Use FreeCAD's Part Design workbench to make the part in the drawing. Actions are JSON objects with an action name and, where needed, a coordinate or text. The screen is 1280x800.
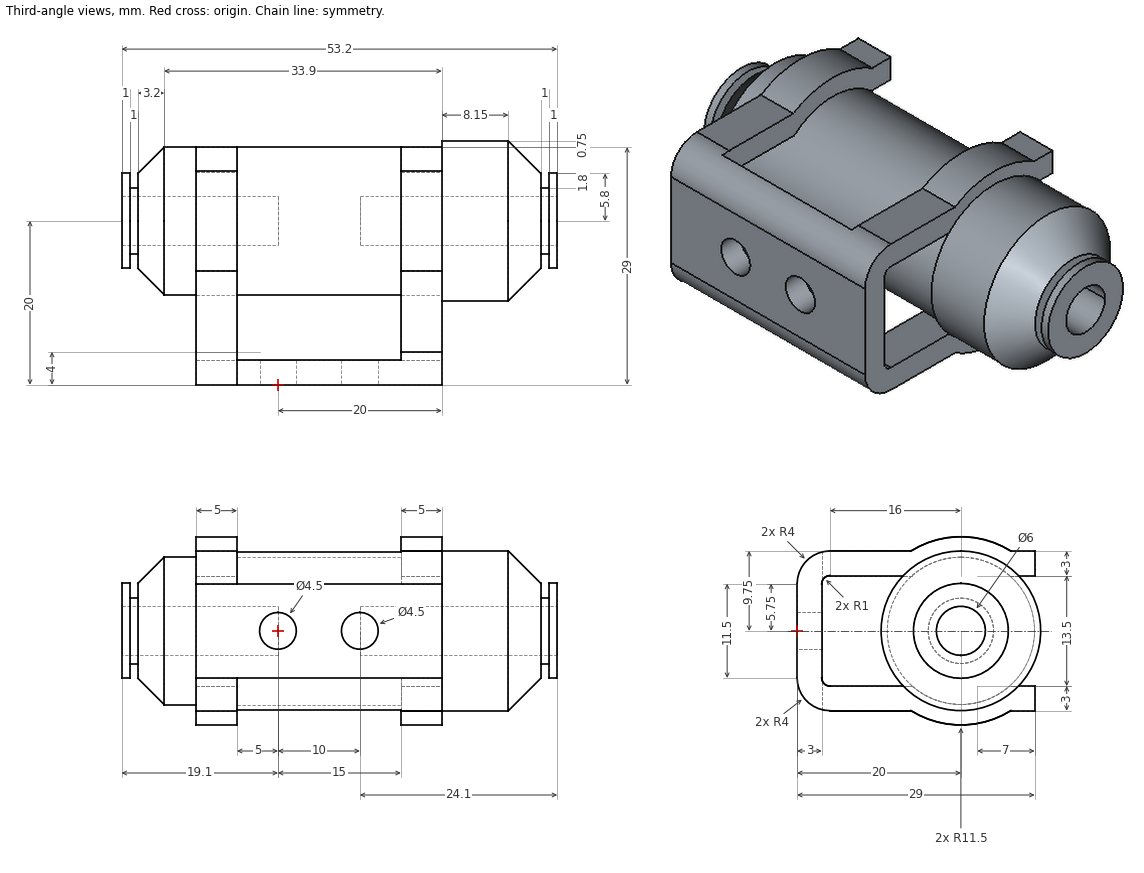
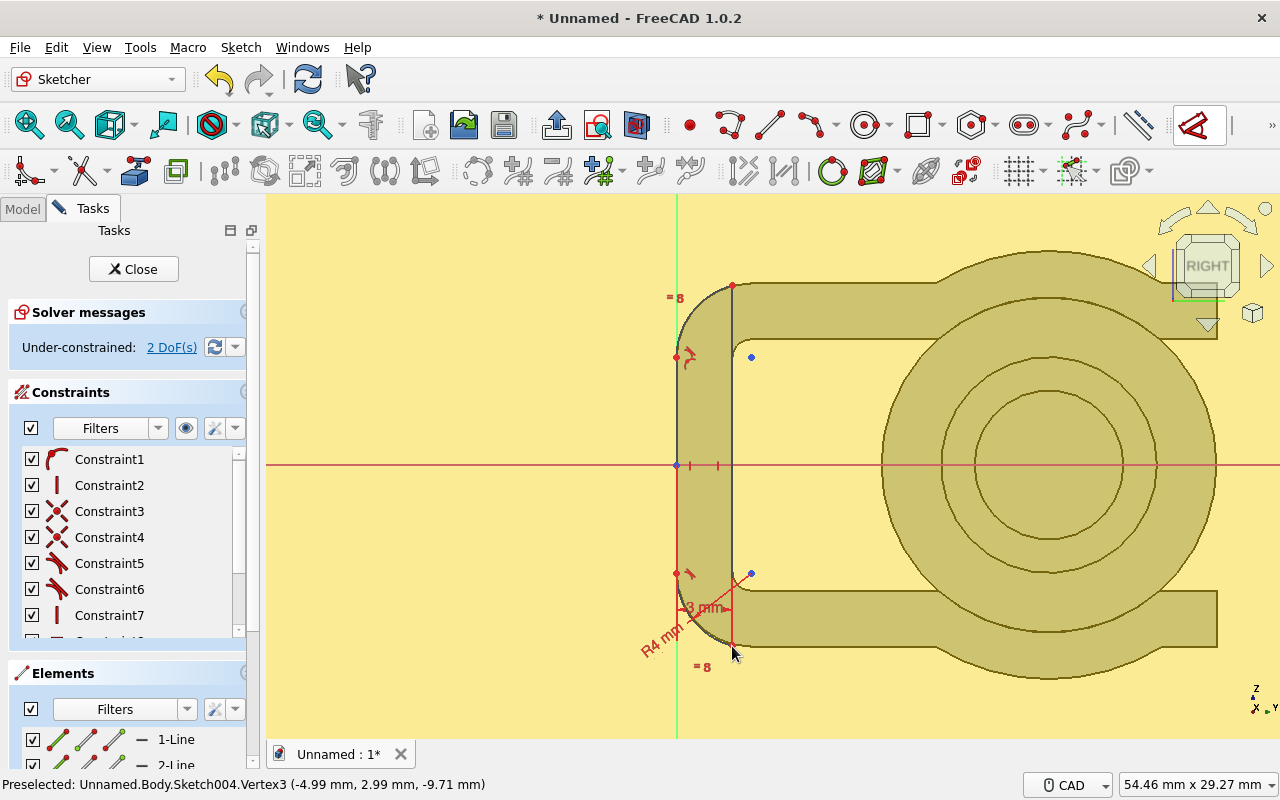
{"action": "left_click", "coordinate": [677, 423]}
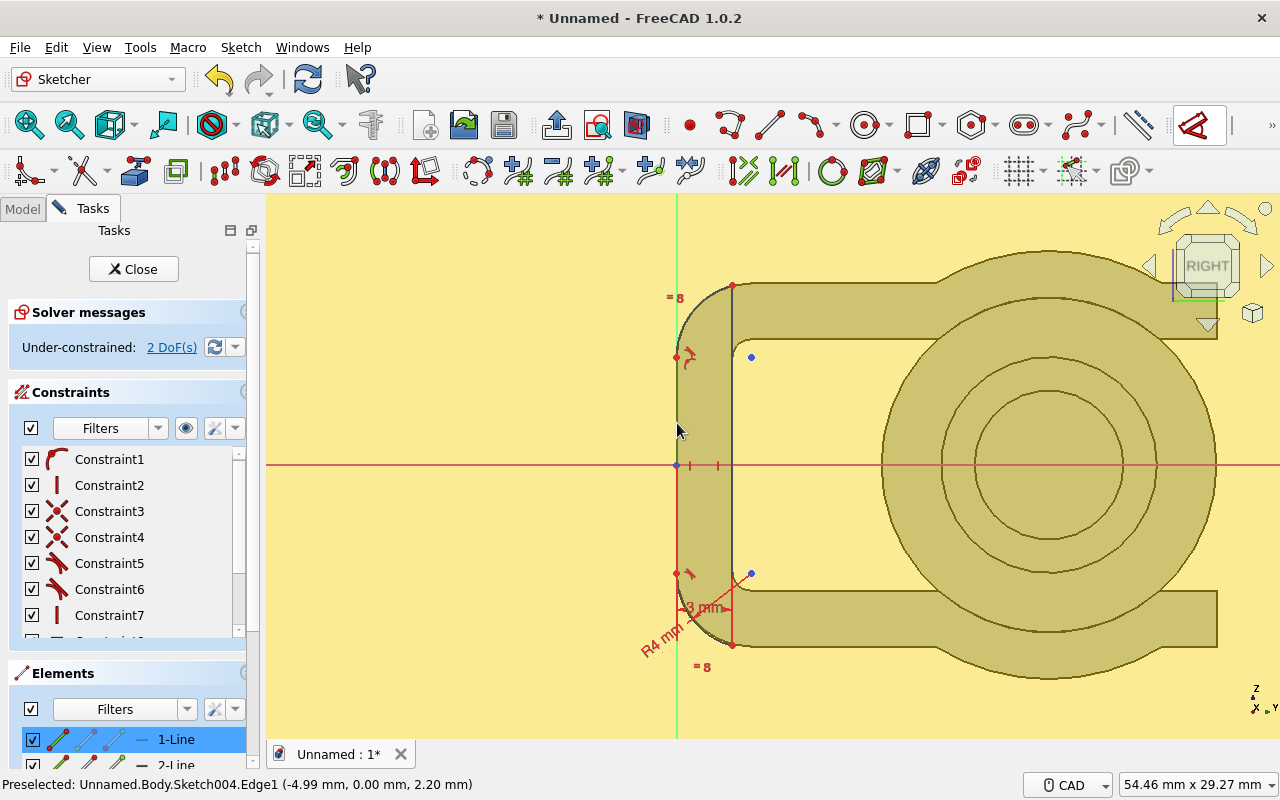
{"action": "left_click", "coordinate": [1220, 126]}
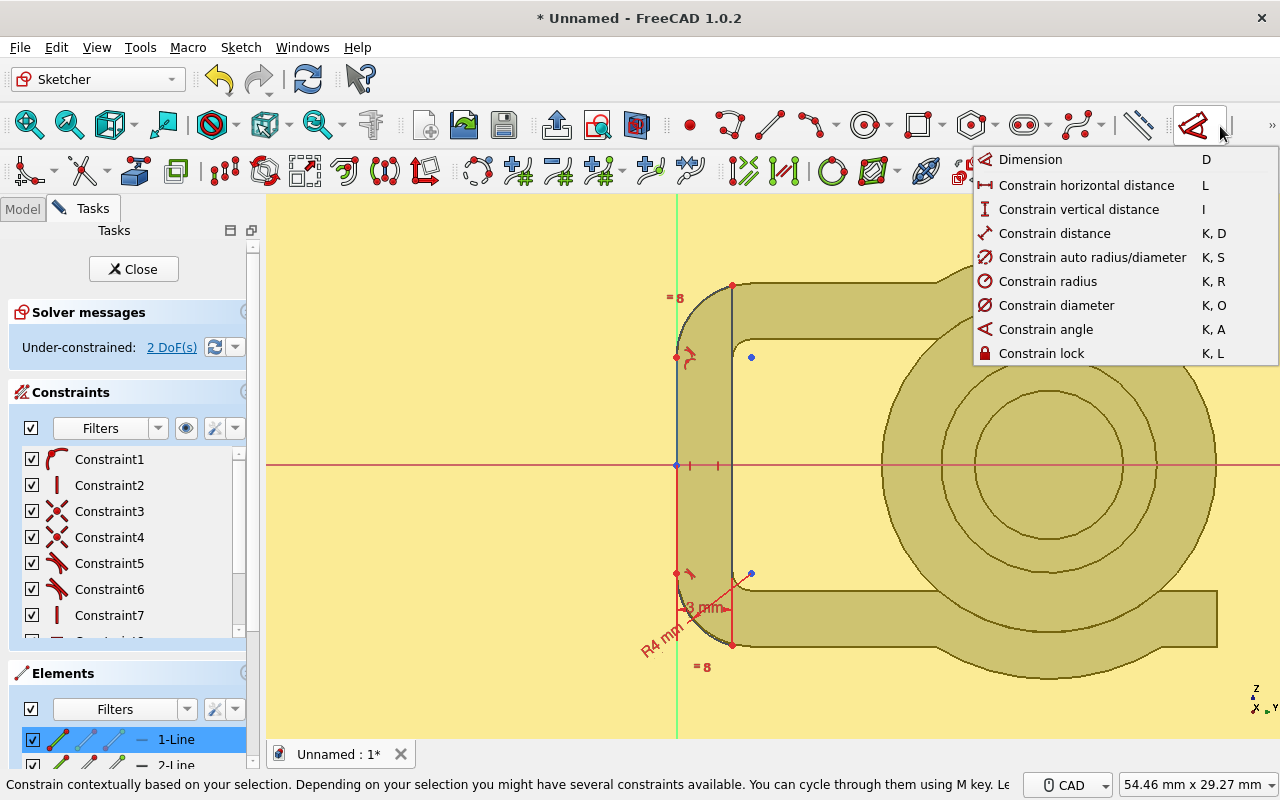
{"action": "left_click", "coordinate": [1126, 209]}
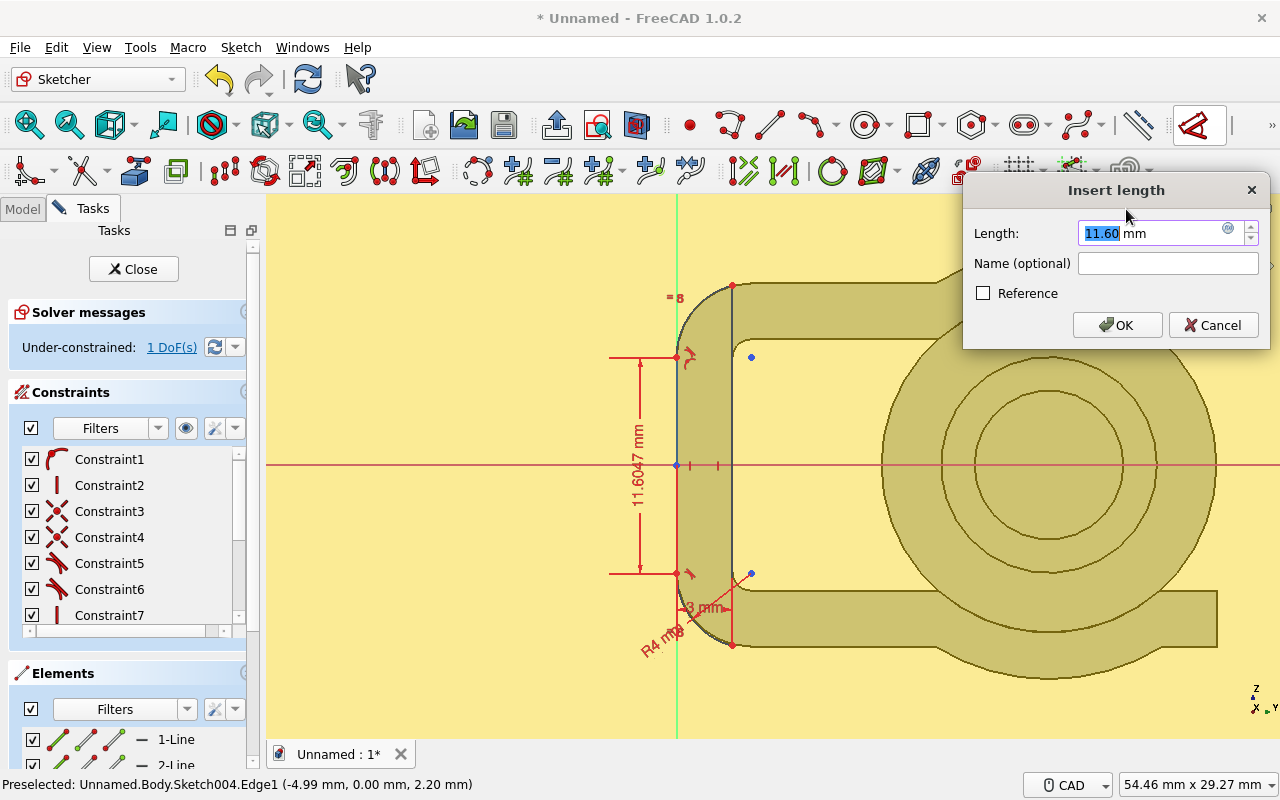
{"action": "type", "text": "11.5"}
{"action": "key", "text": "Return"}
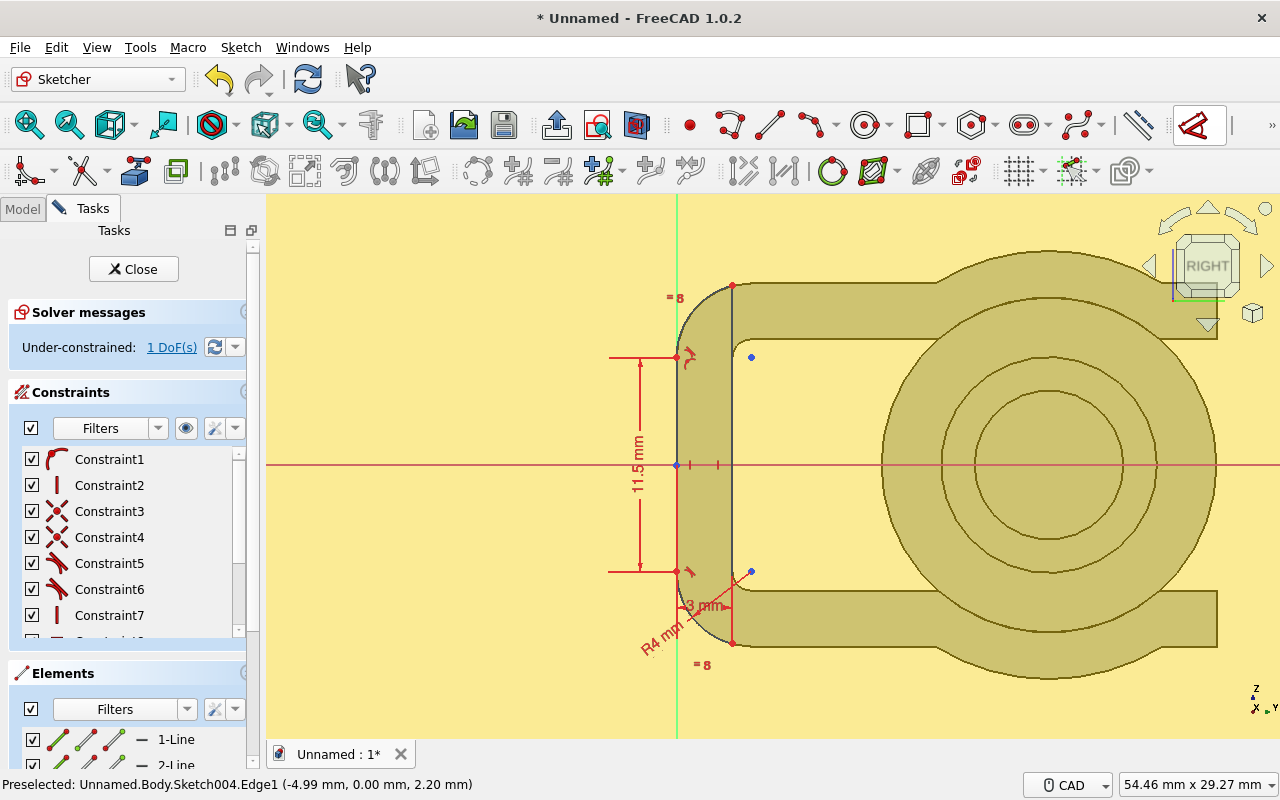
{"action": "left_click", "coordinate": [677, 358]}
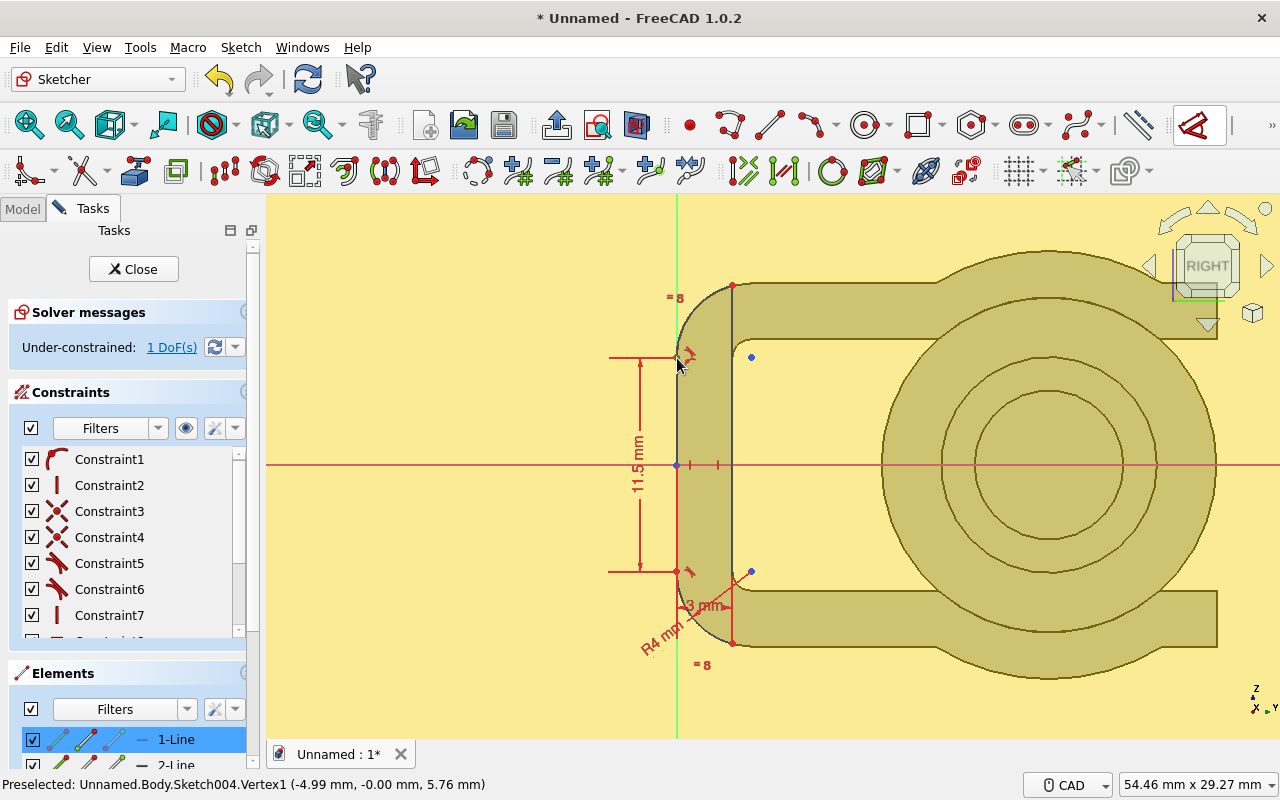
{"action": "left_click", "coordinate": [1220, 126]}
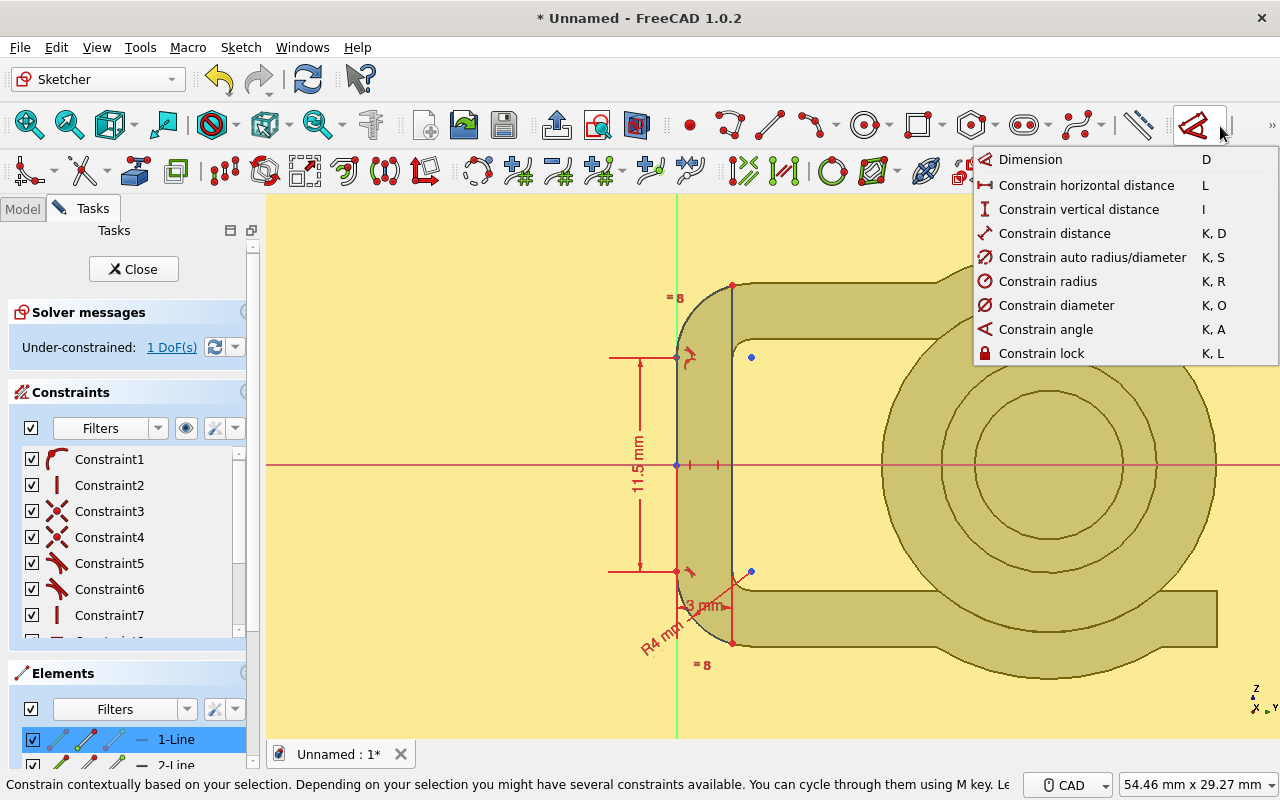
{"action": "left_click", "coordinate": [1126, 209]}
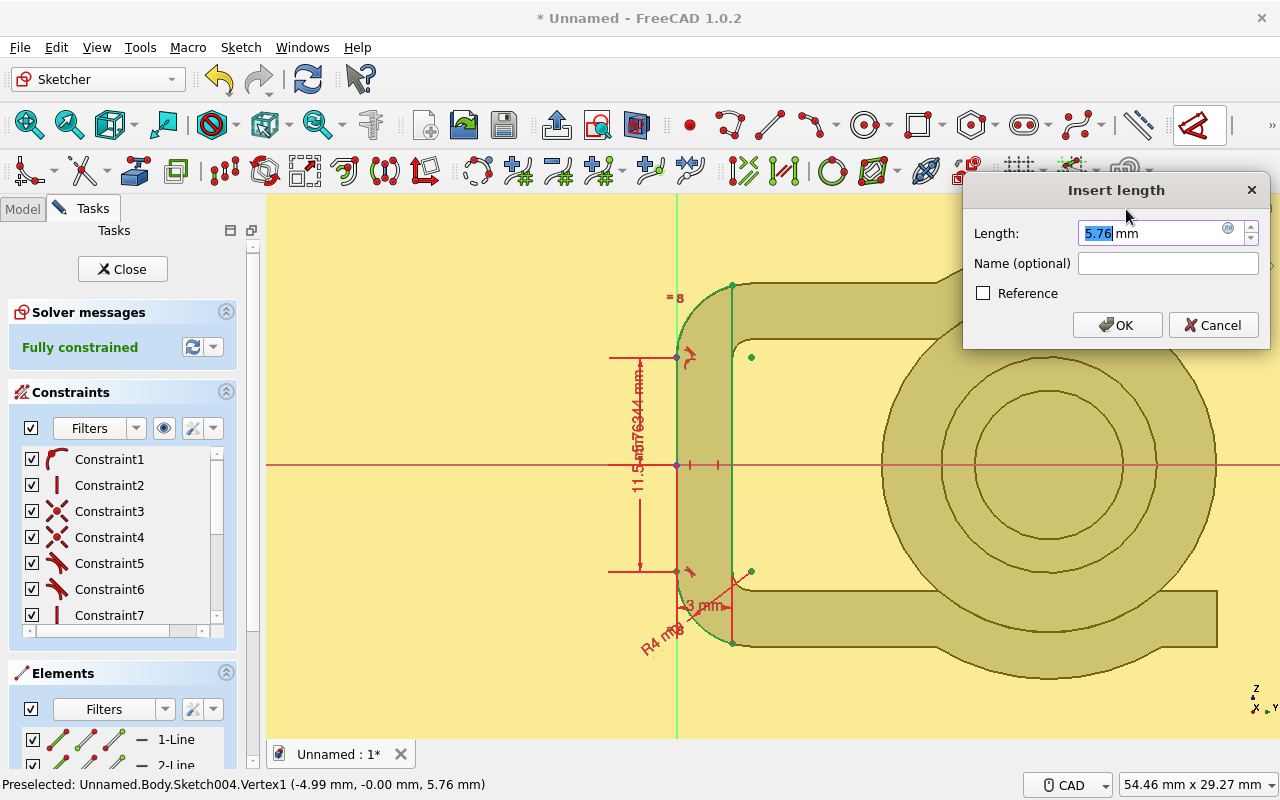
{"action": "type", "text": "5.75"}
{"action": "key", "text": "Return"}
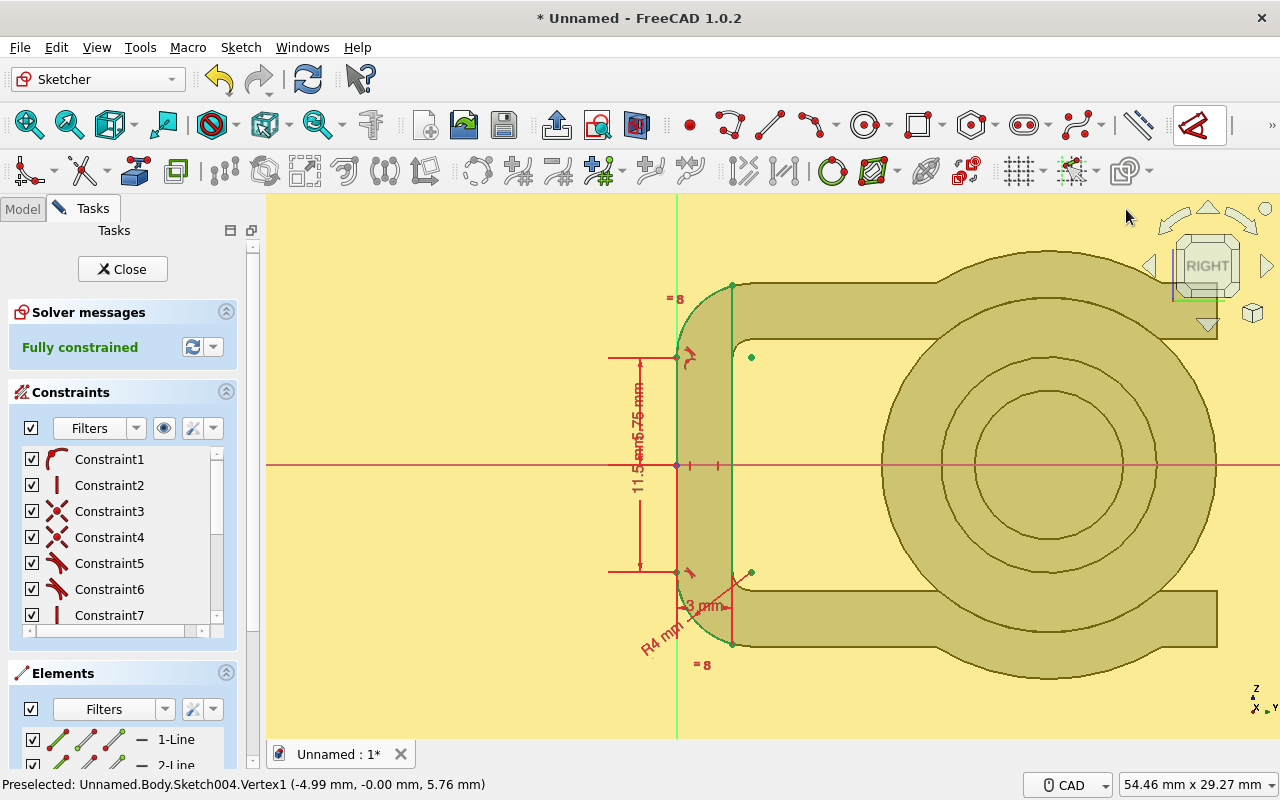
{"action": "left_click", "coordinate": [123, 269]}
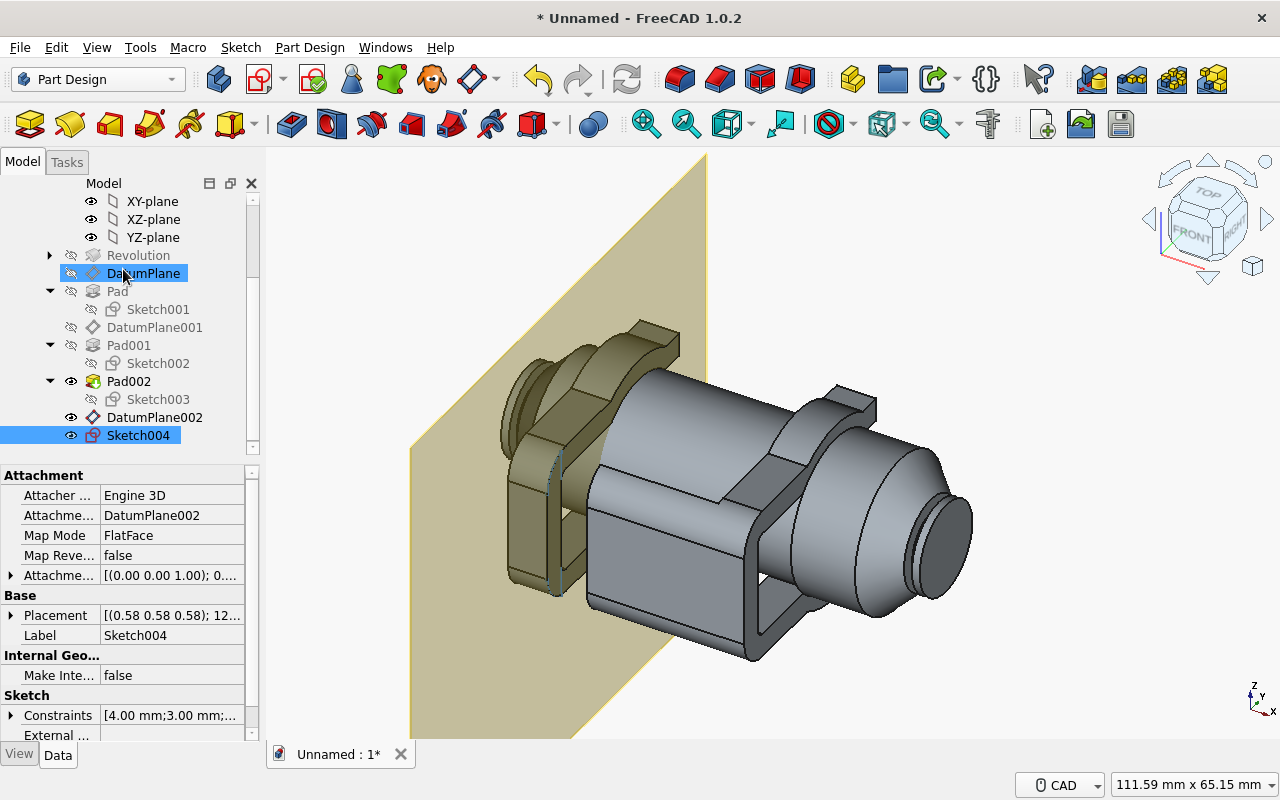
{"action": "left_click", "coordinate": [30, 124]}